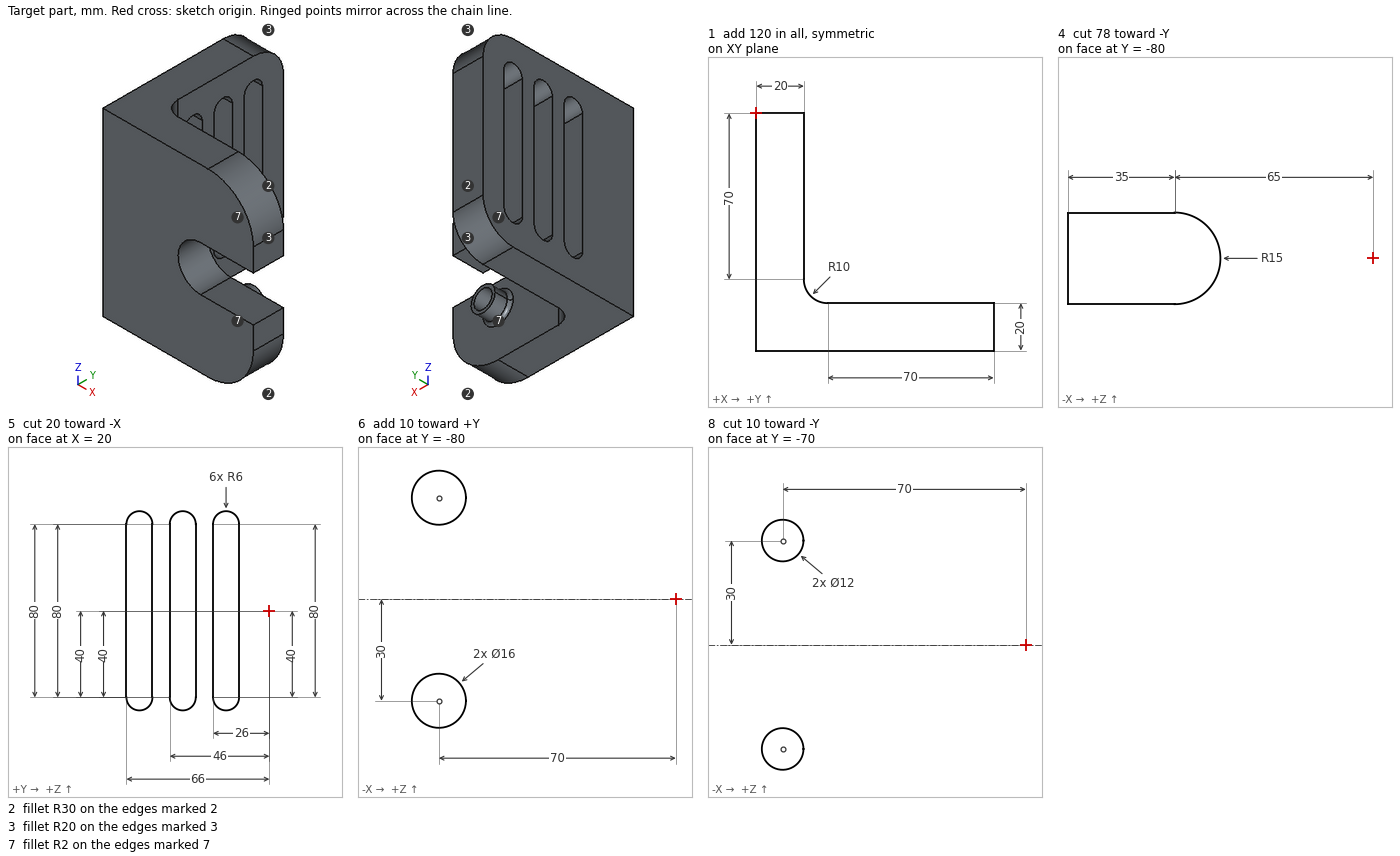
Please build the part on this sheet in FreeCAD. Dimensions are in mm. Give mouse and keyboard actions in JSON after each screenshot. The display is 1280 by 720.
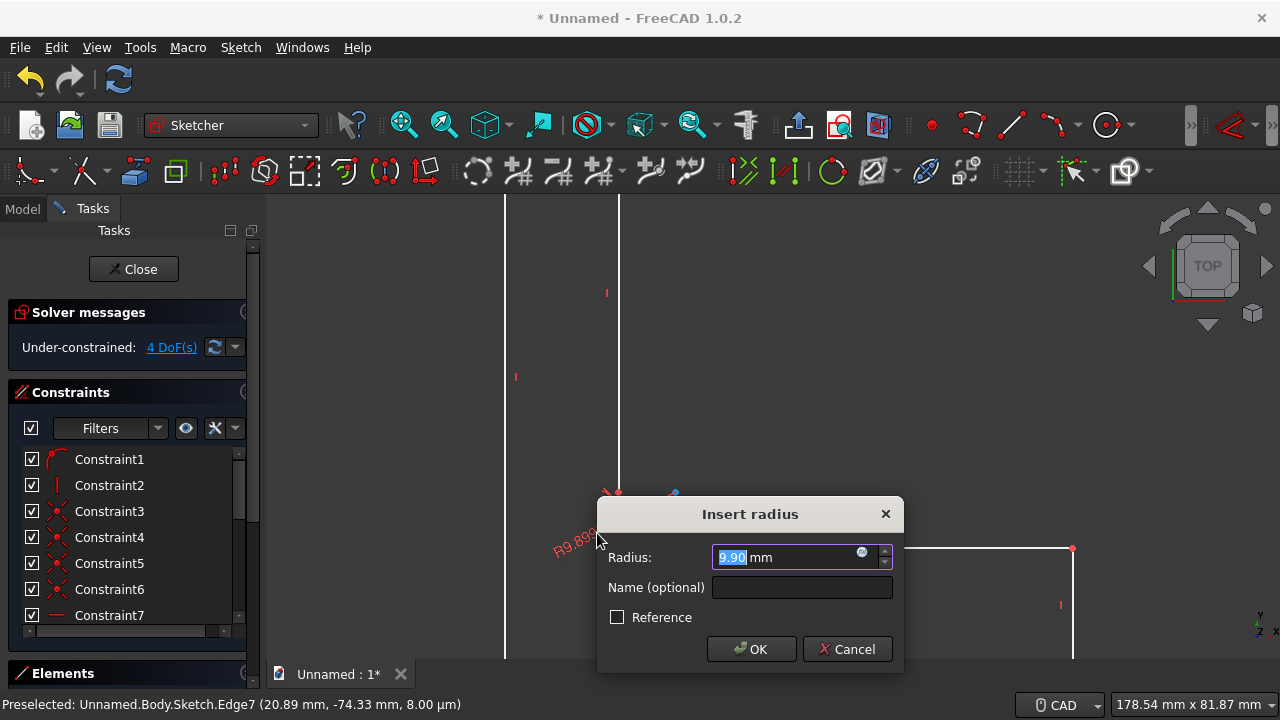
{"action": "type", "text": "10"}
{"action": "key", "text": "Return"}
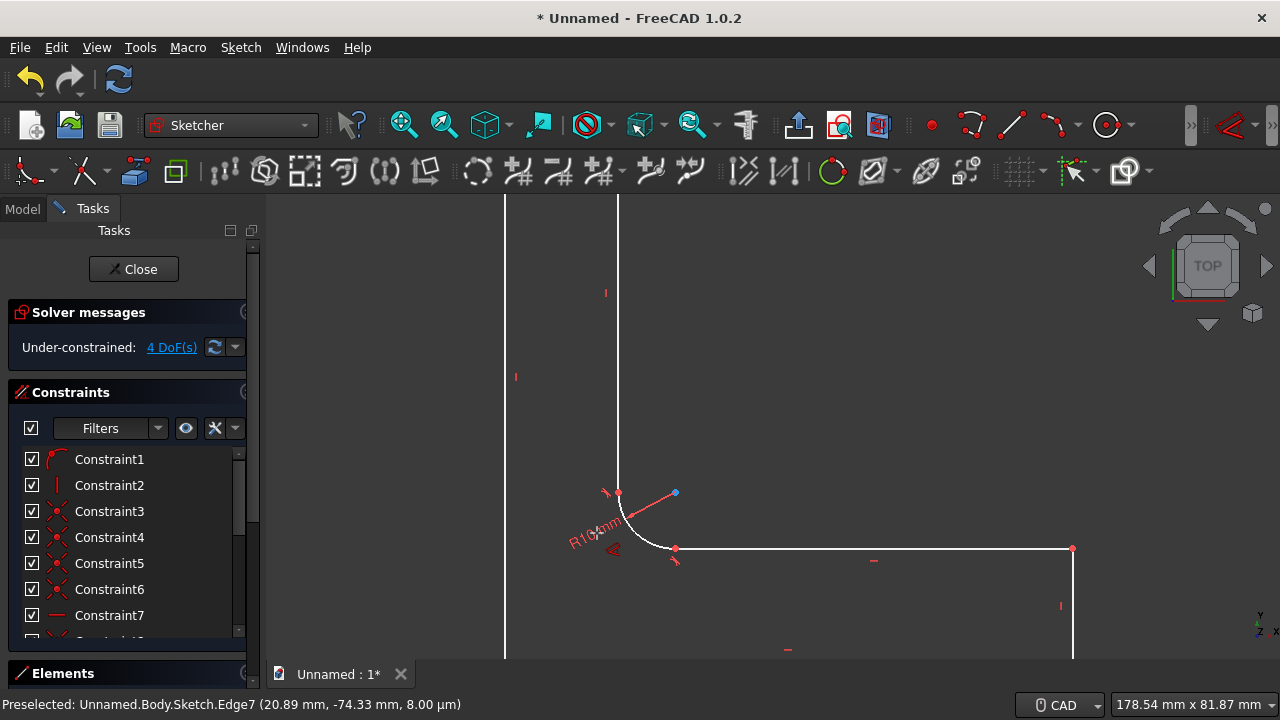
{"action": "left_click", "coordinate": [618, 372]}
{"action": "left_click", "coordinate": [584, 357]}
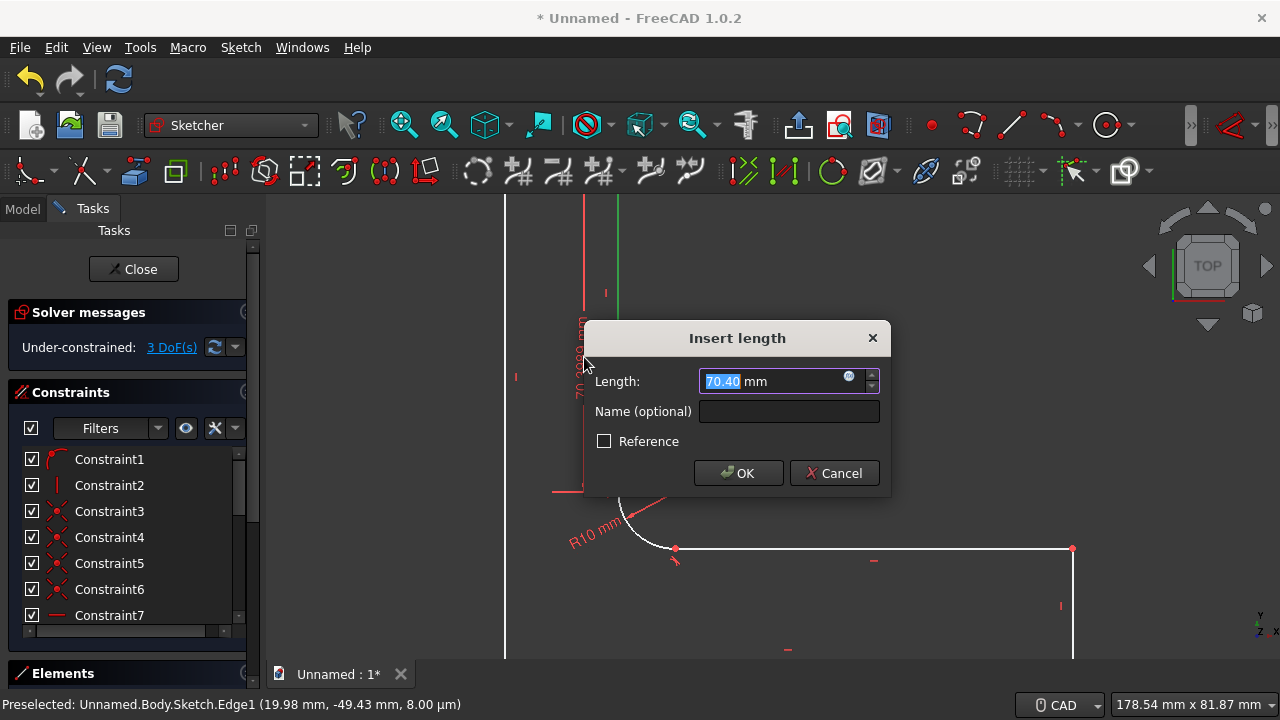
{"action": "type", "text": "70"}
{"action": "key", "text": "Return"}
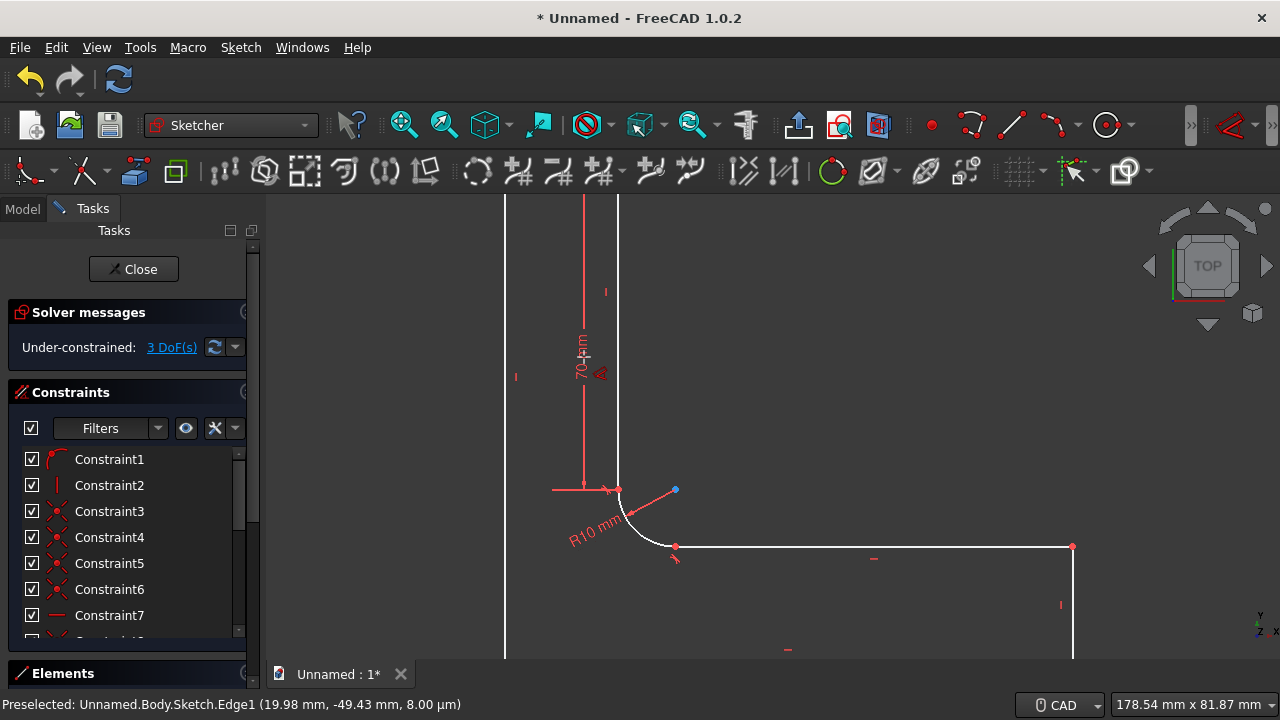
{"action": "scroll", "coordinate": [602, 488], "scroll_direction": "down", "scroll_amount": 3}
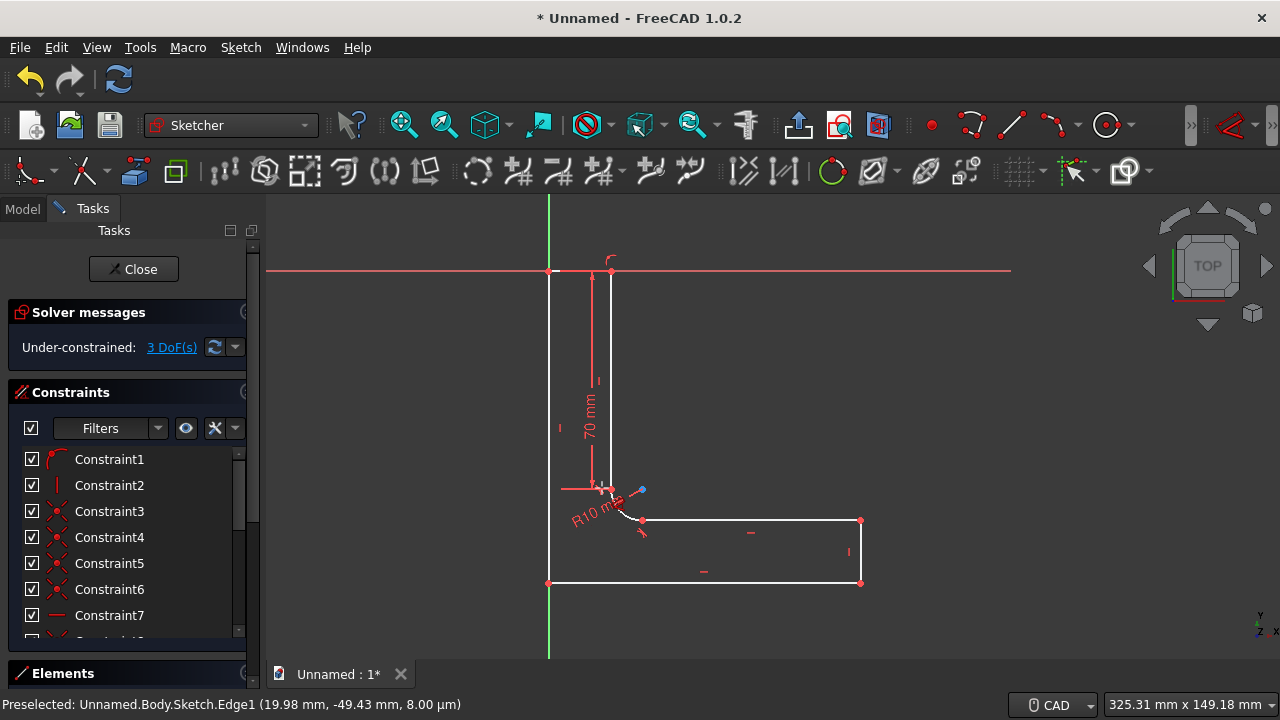
{"action": "left_click", "coordinate": [592, 271]}
{"action": "left_click", "coordinate": [580, 237]}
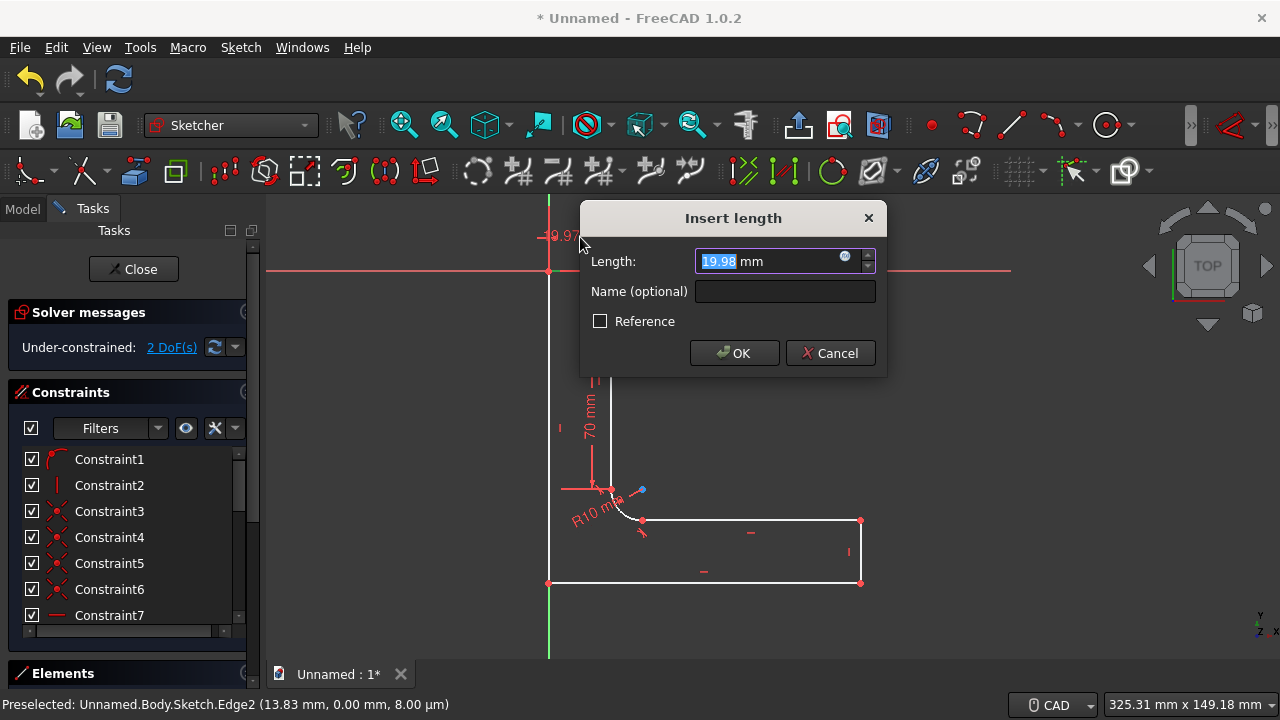
{"action": "type", "text": "20"}
{"action": "key", "text": "Return"}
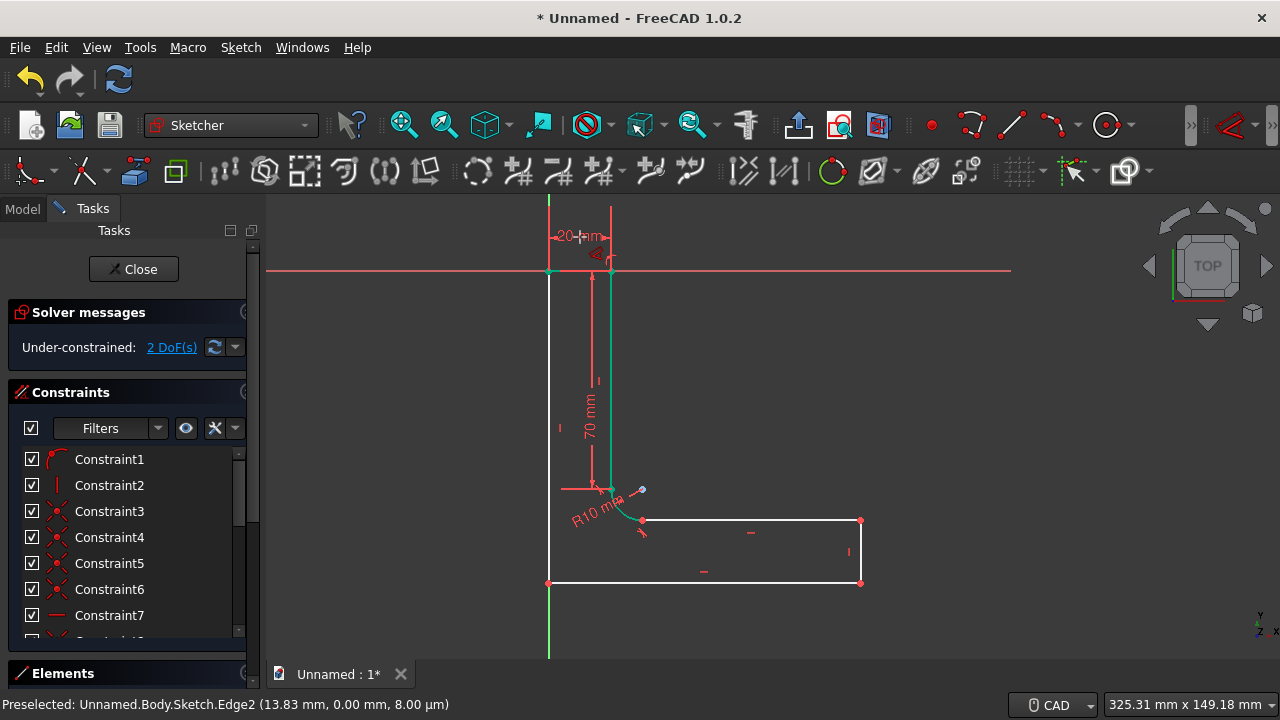
{"action": "left_click", "coordinate": [861, 565]}
{"action": "left_click", "coordinate": [895, 552]}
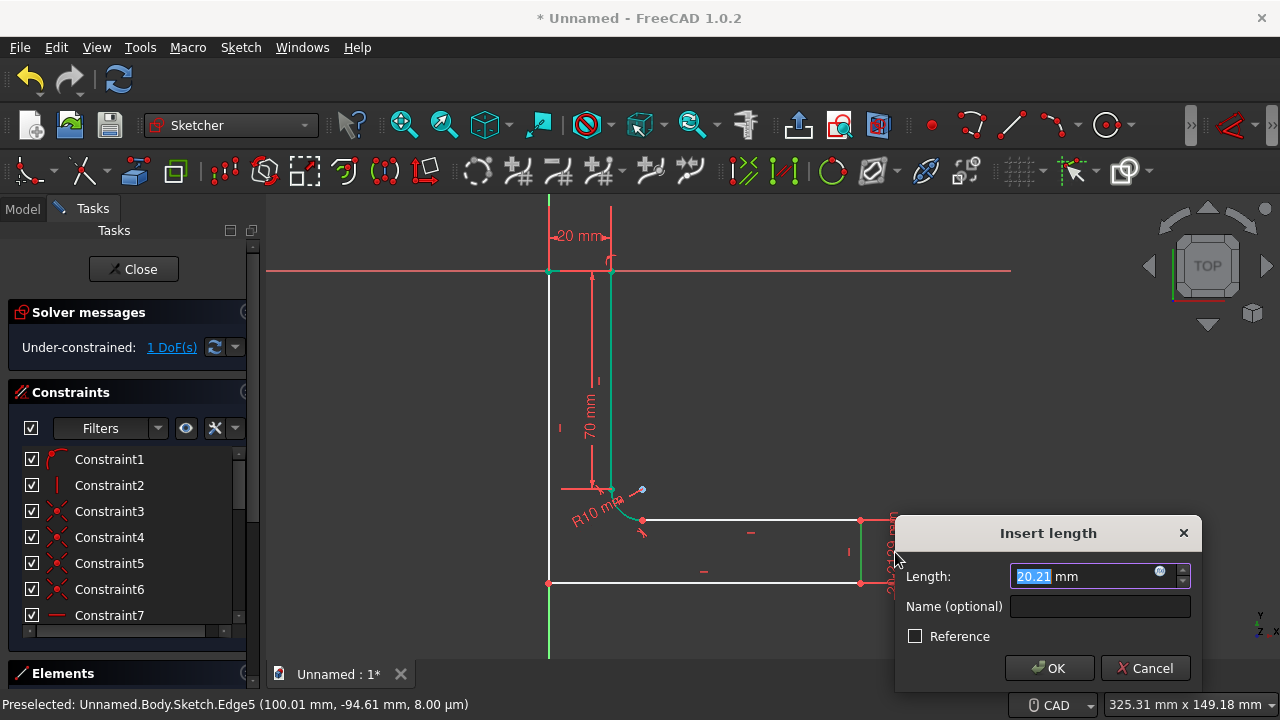
{"action": "type", "text": "20"}
{"action": "key", "text": "Return"}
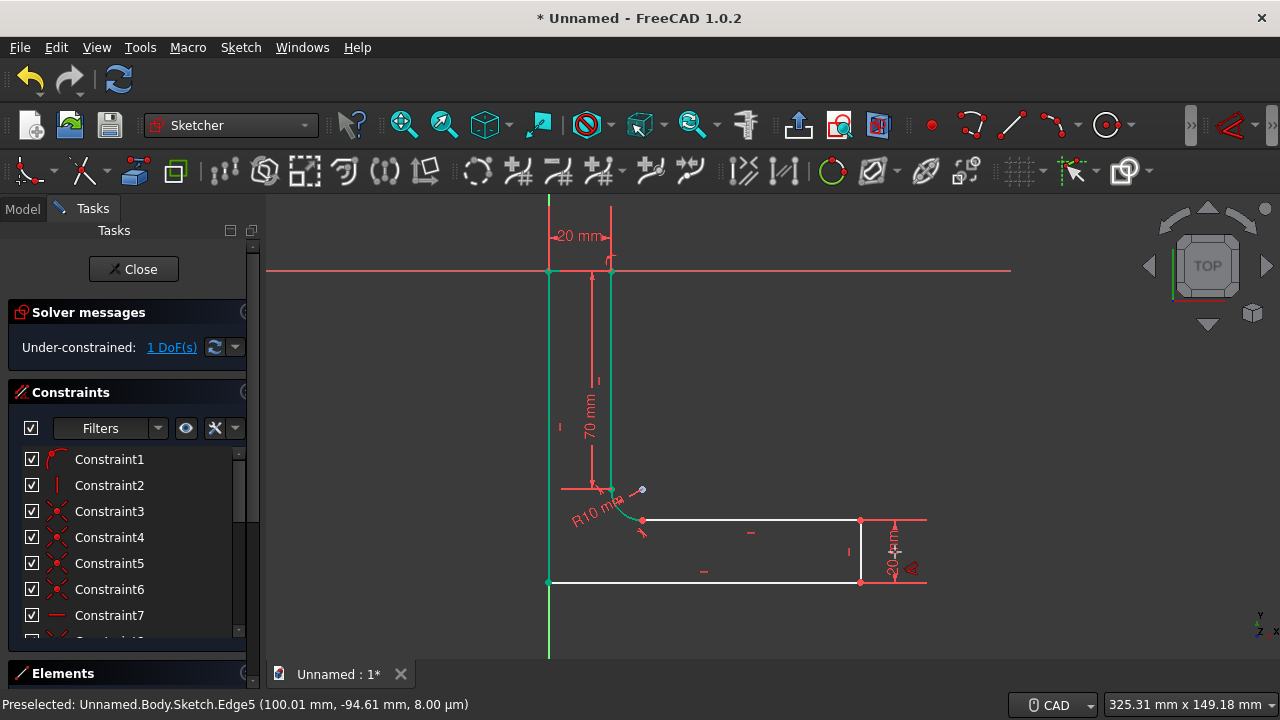
{"action": "left_click", "coordinate": [795, 520]}
{"action": "left_click", "coordinate": [752, 554]}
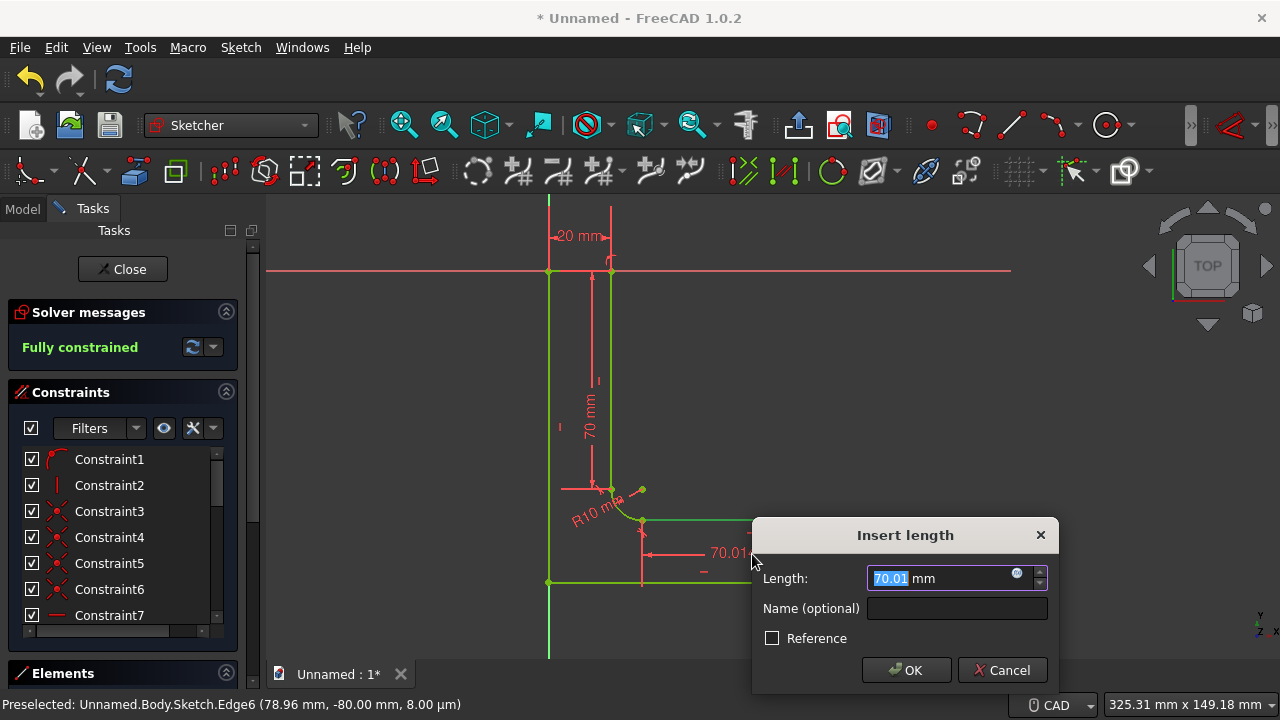
{"action": "type", "text": "70"}
{"action": "key", "text": "Return"}
{"action": "key", "text": "Escape"}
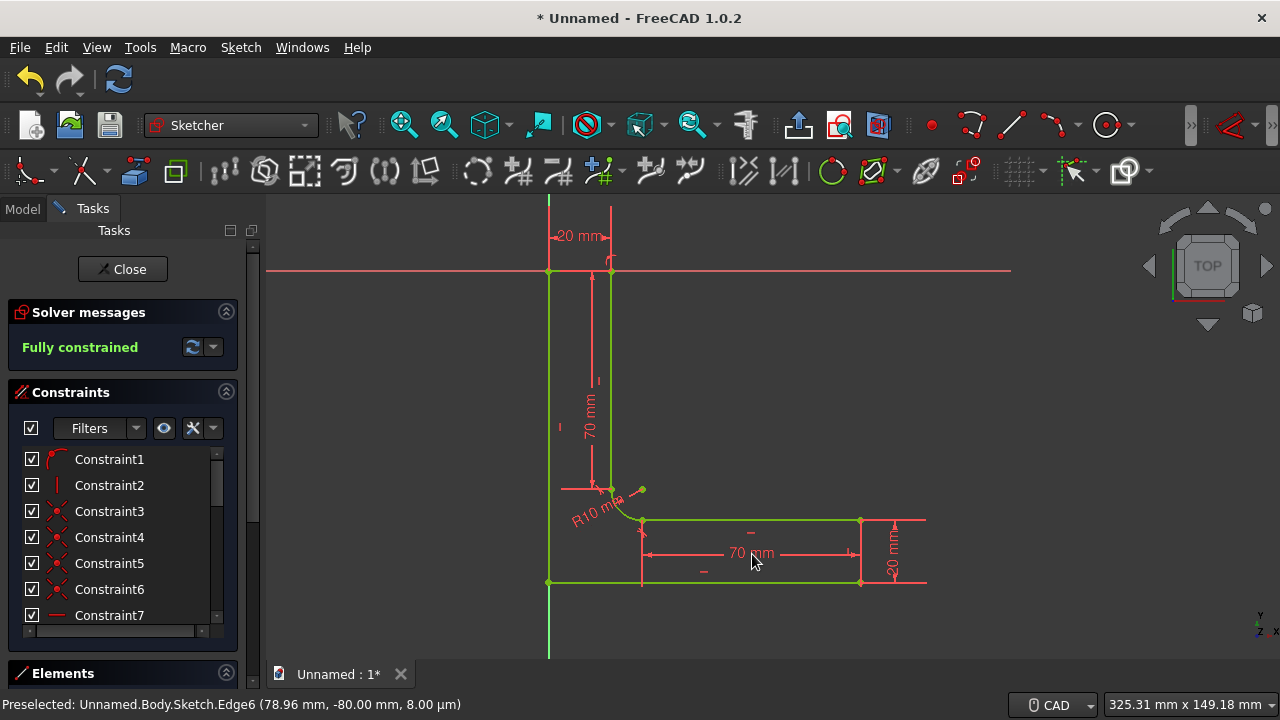
{"action": "left_click", "coordinate": [123, 269]}